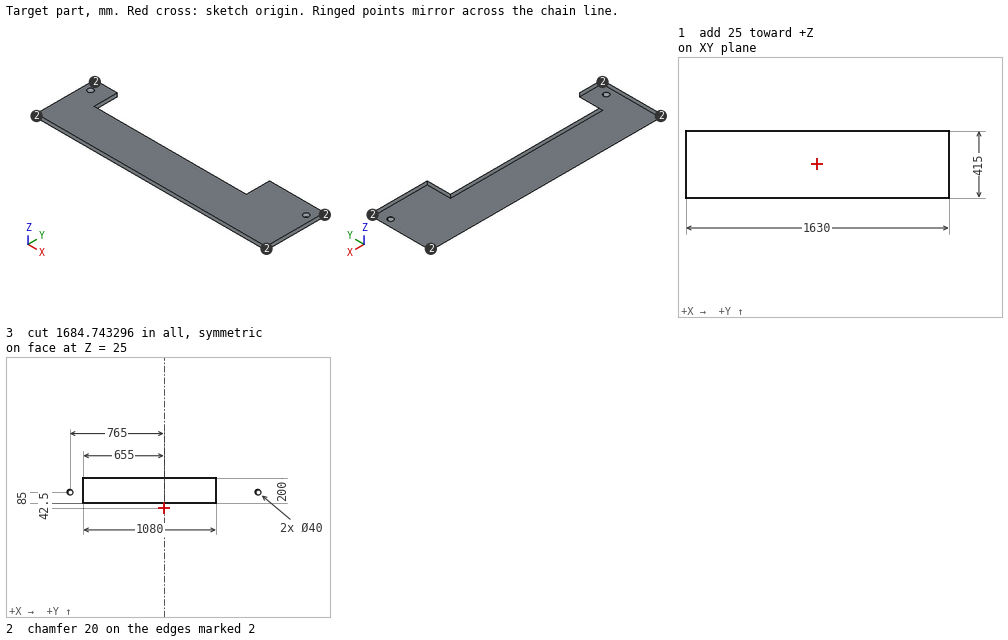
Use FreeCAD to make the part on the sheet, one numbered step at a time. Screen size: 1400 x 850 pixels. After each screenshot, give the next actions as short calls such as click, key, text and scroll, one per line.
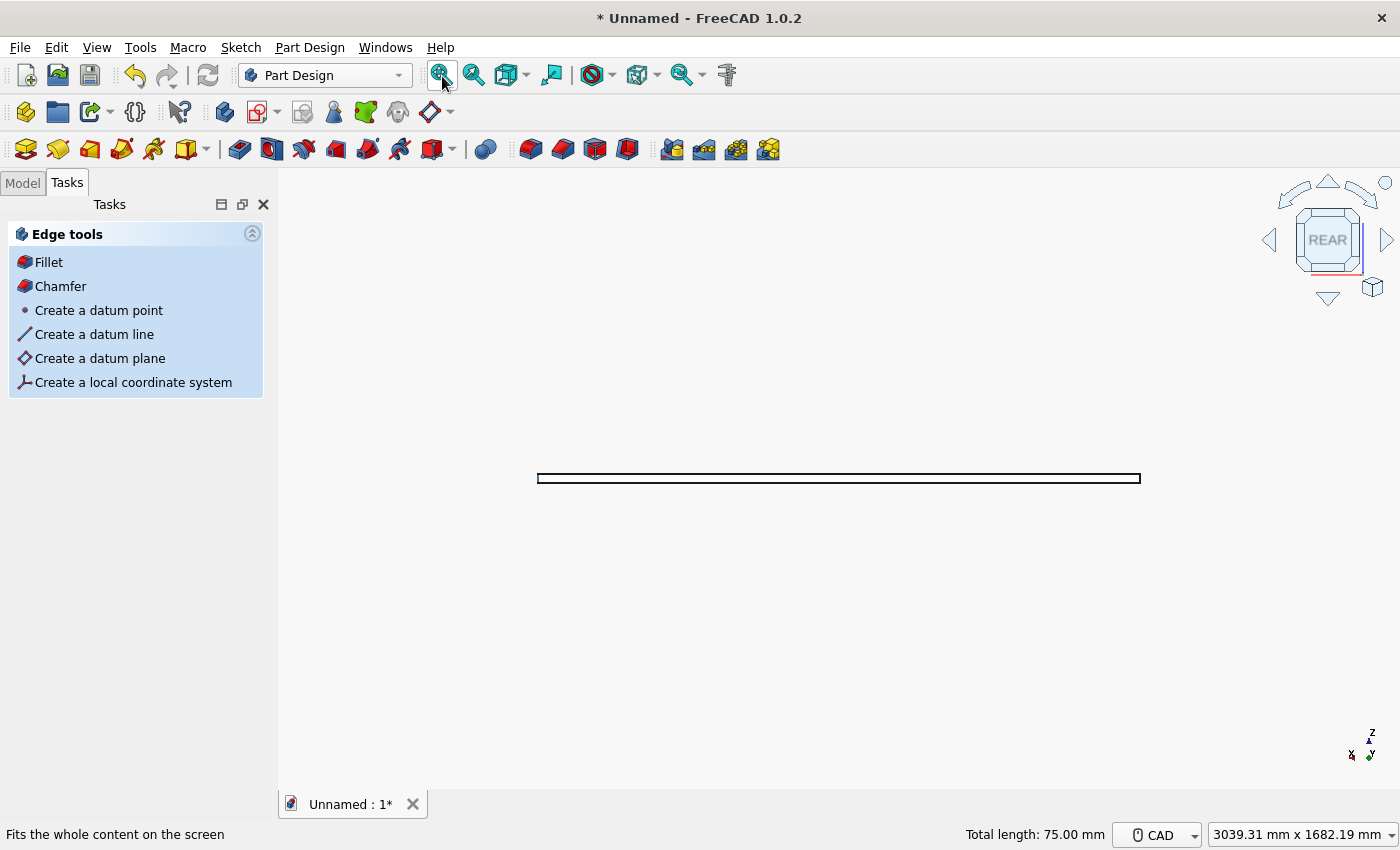
scroll(1140, 478, up, 8)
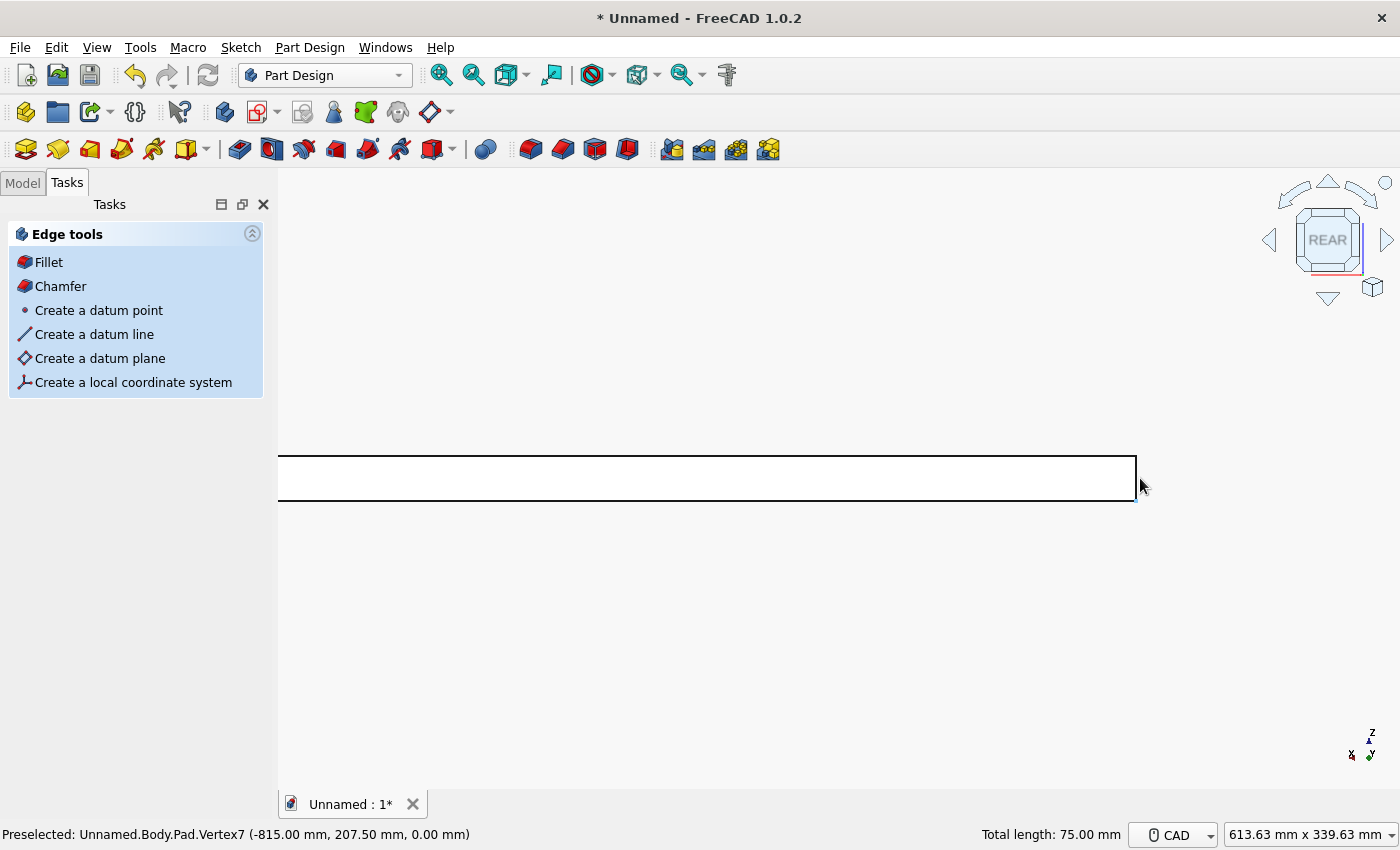
click(1136, 478, ctrl)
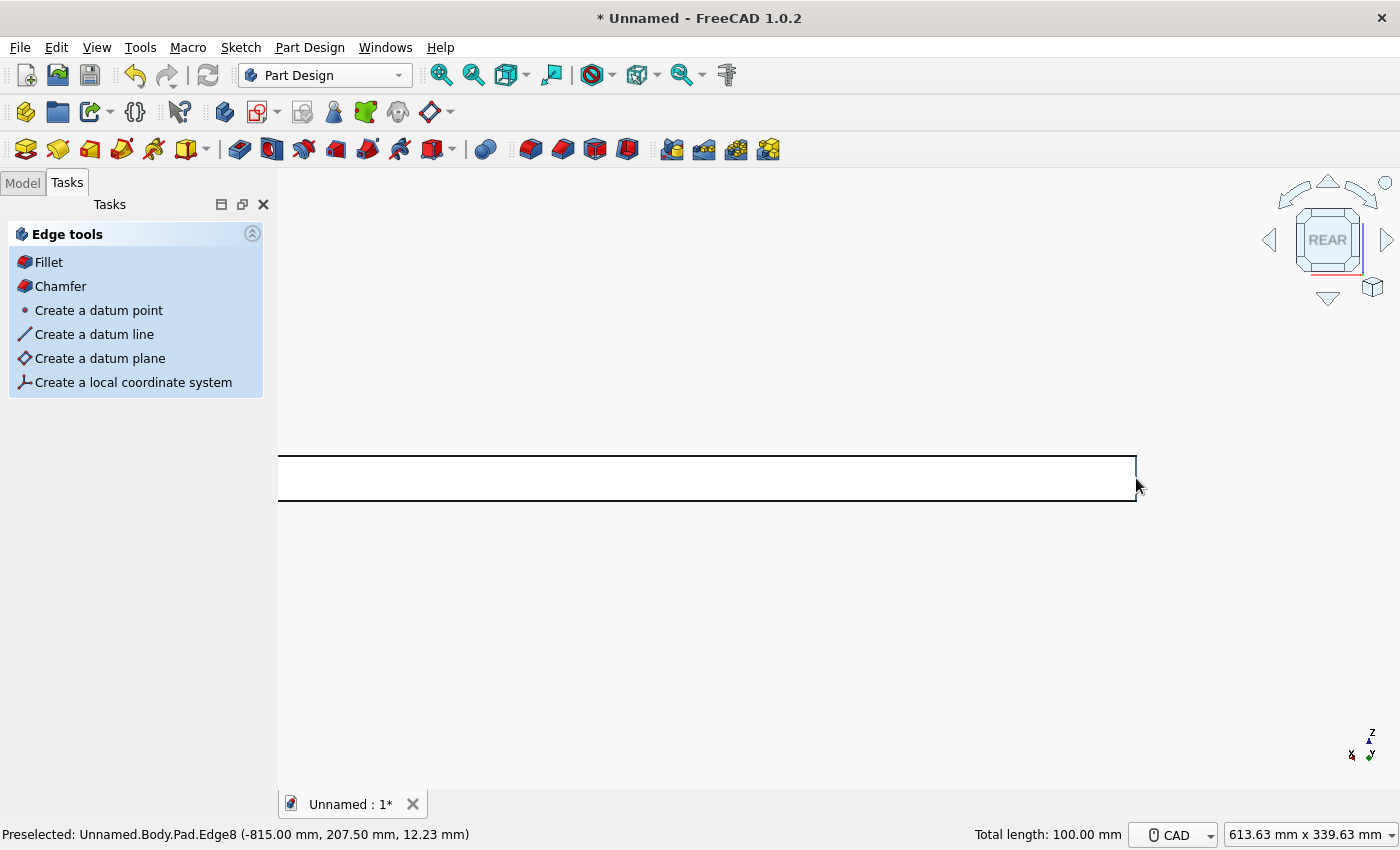
click(564, 150)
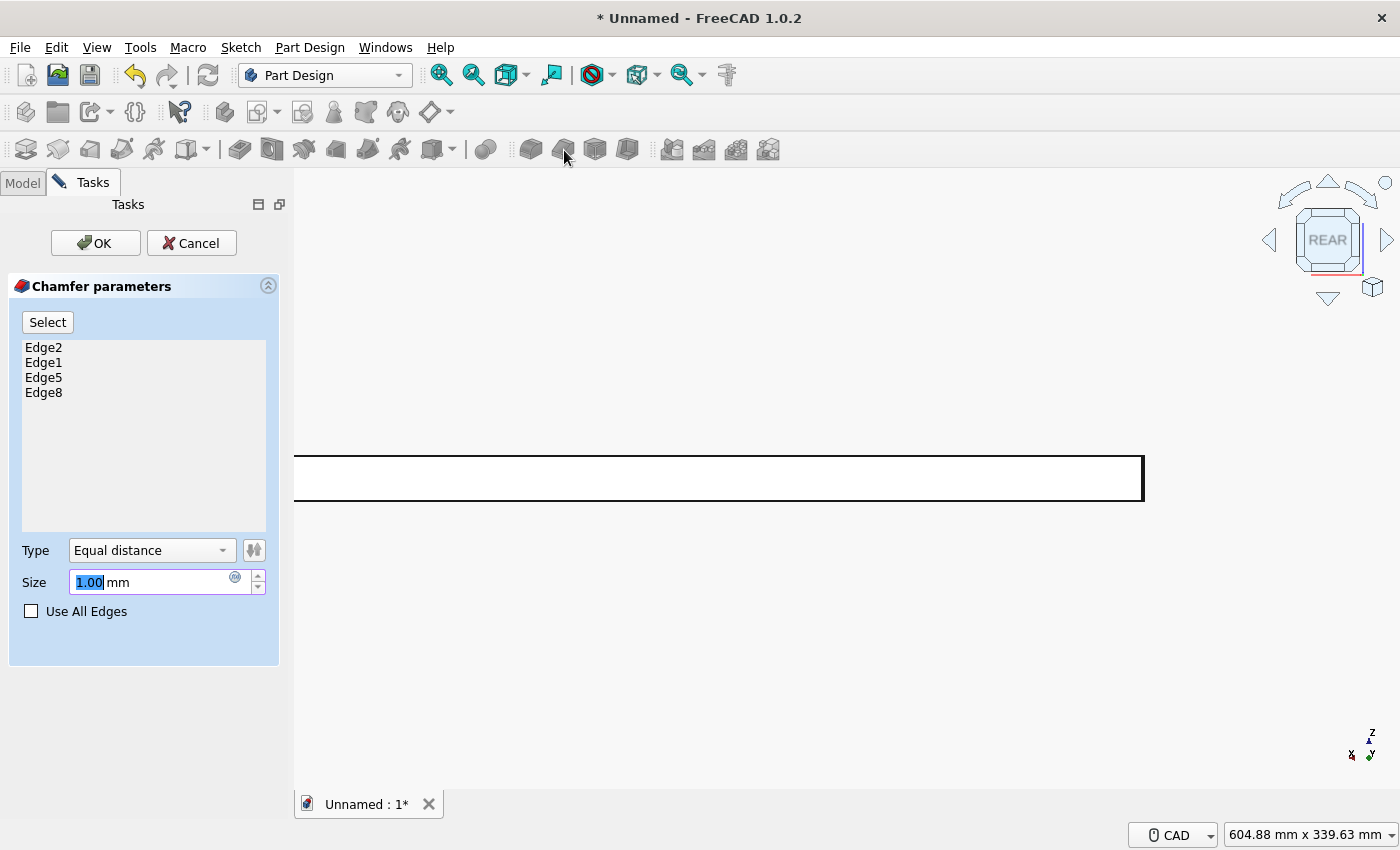
text(20)
key(Tab)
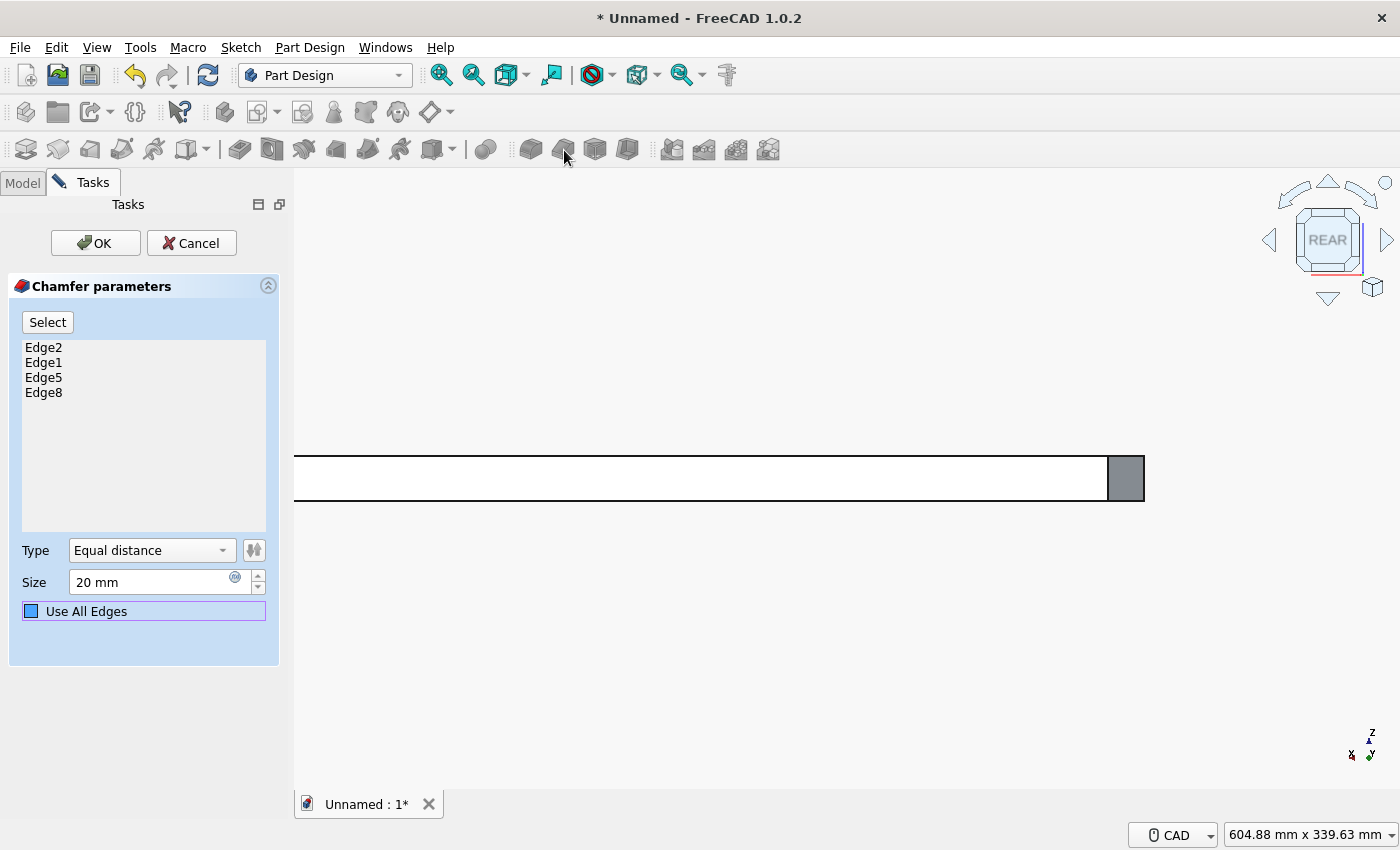
click(96, 243)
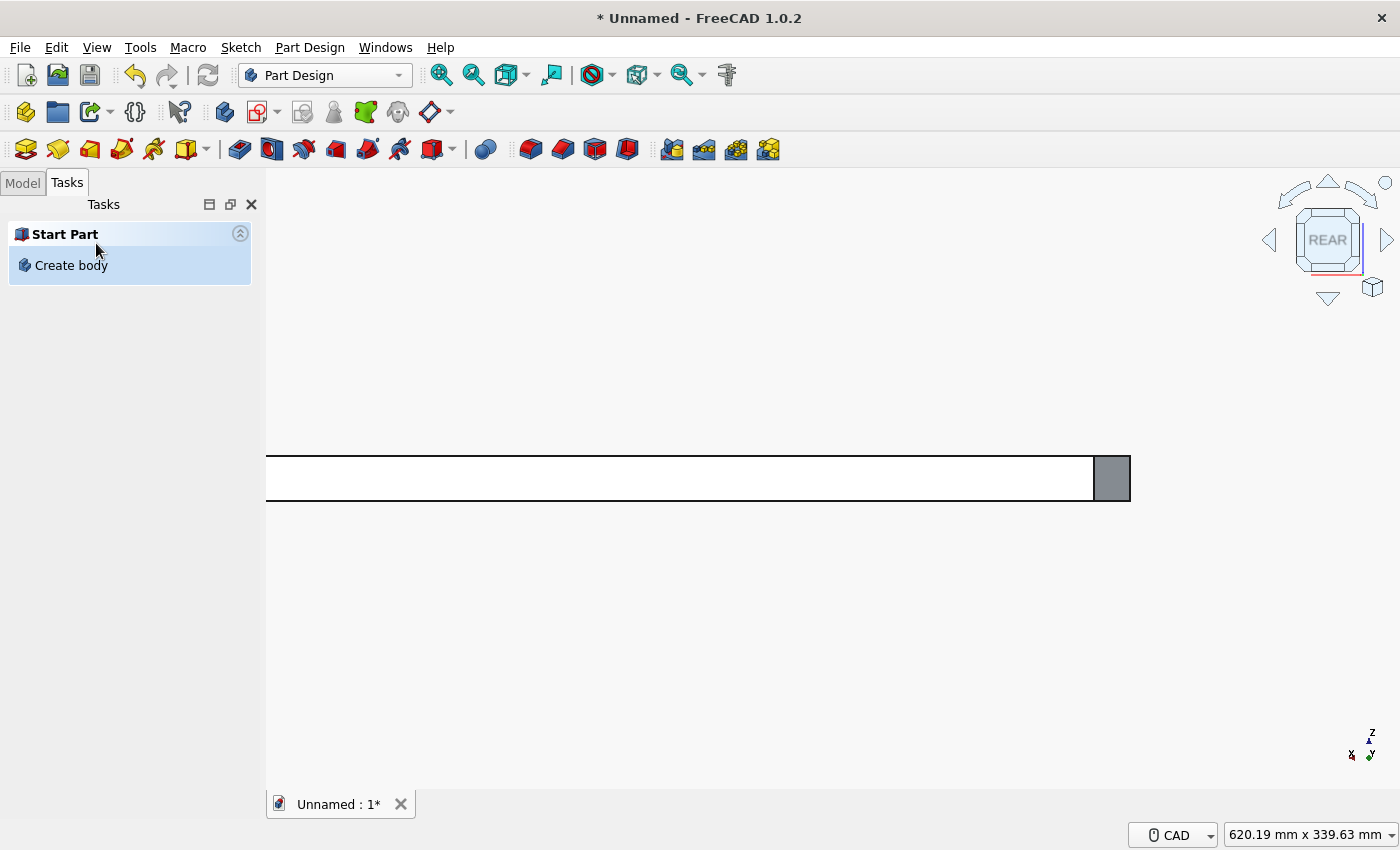
click(442, 76)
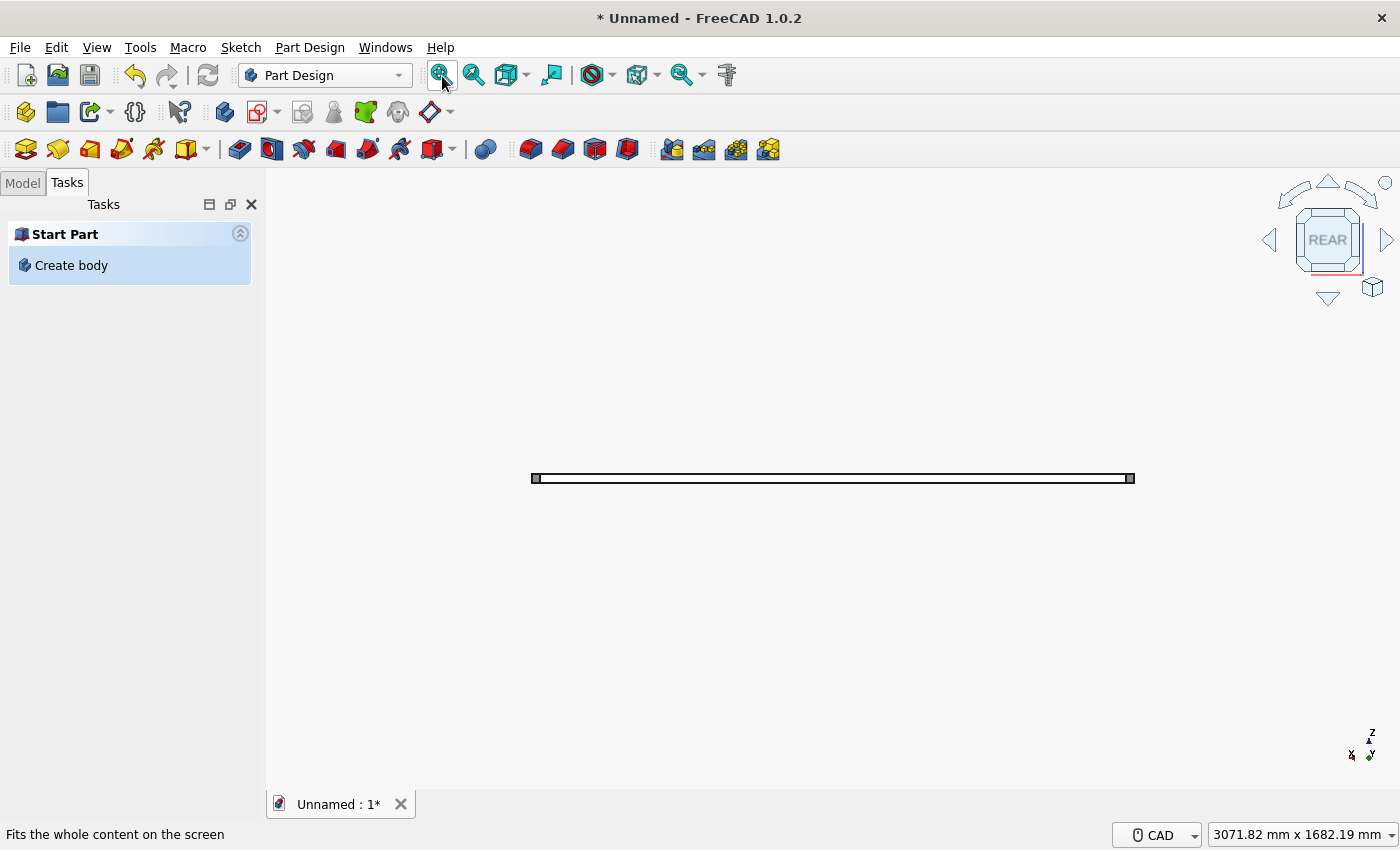
key(0)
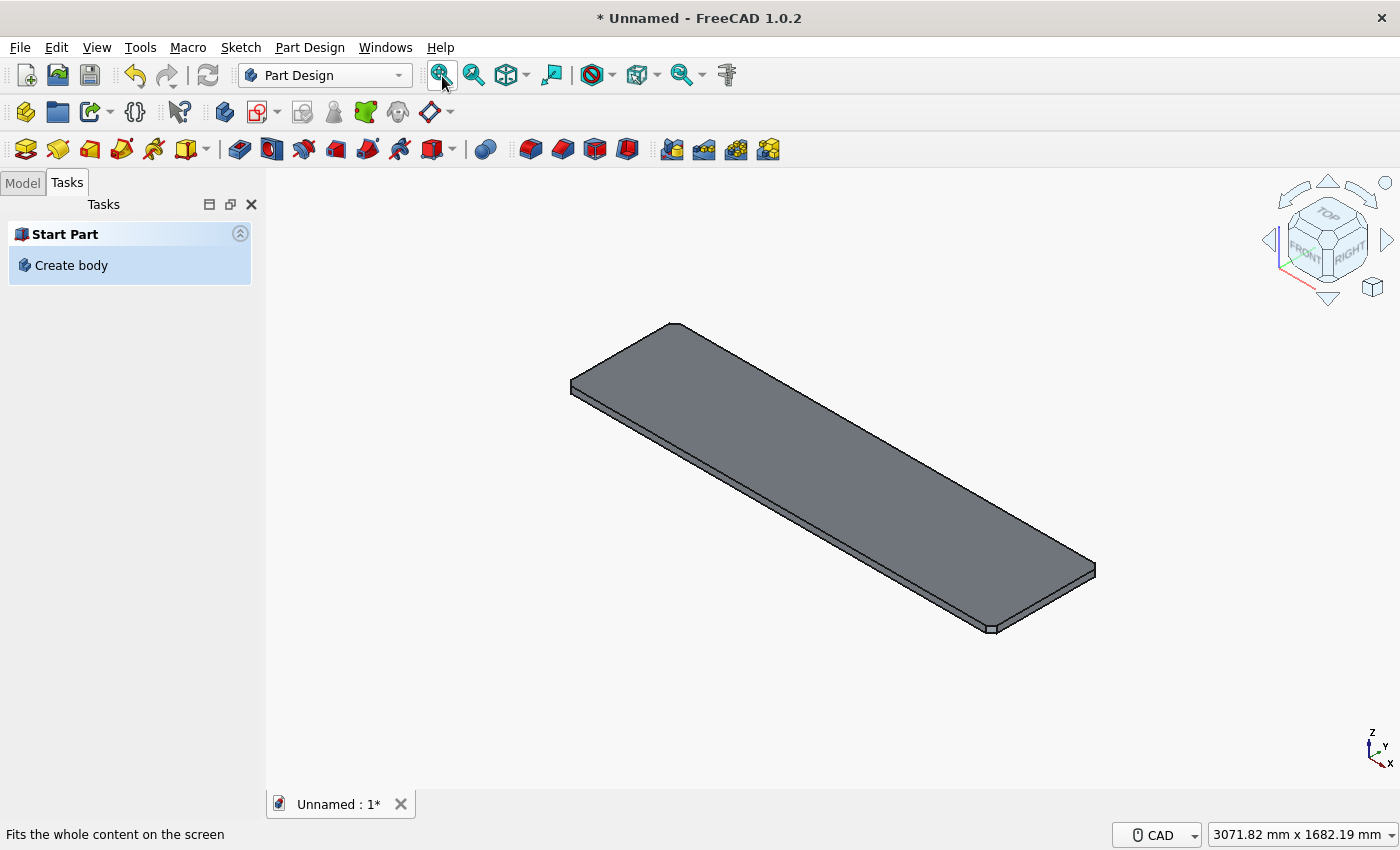
click(955, 544)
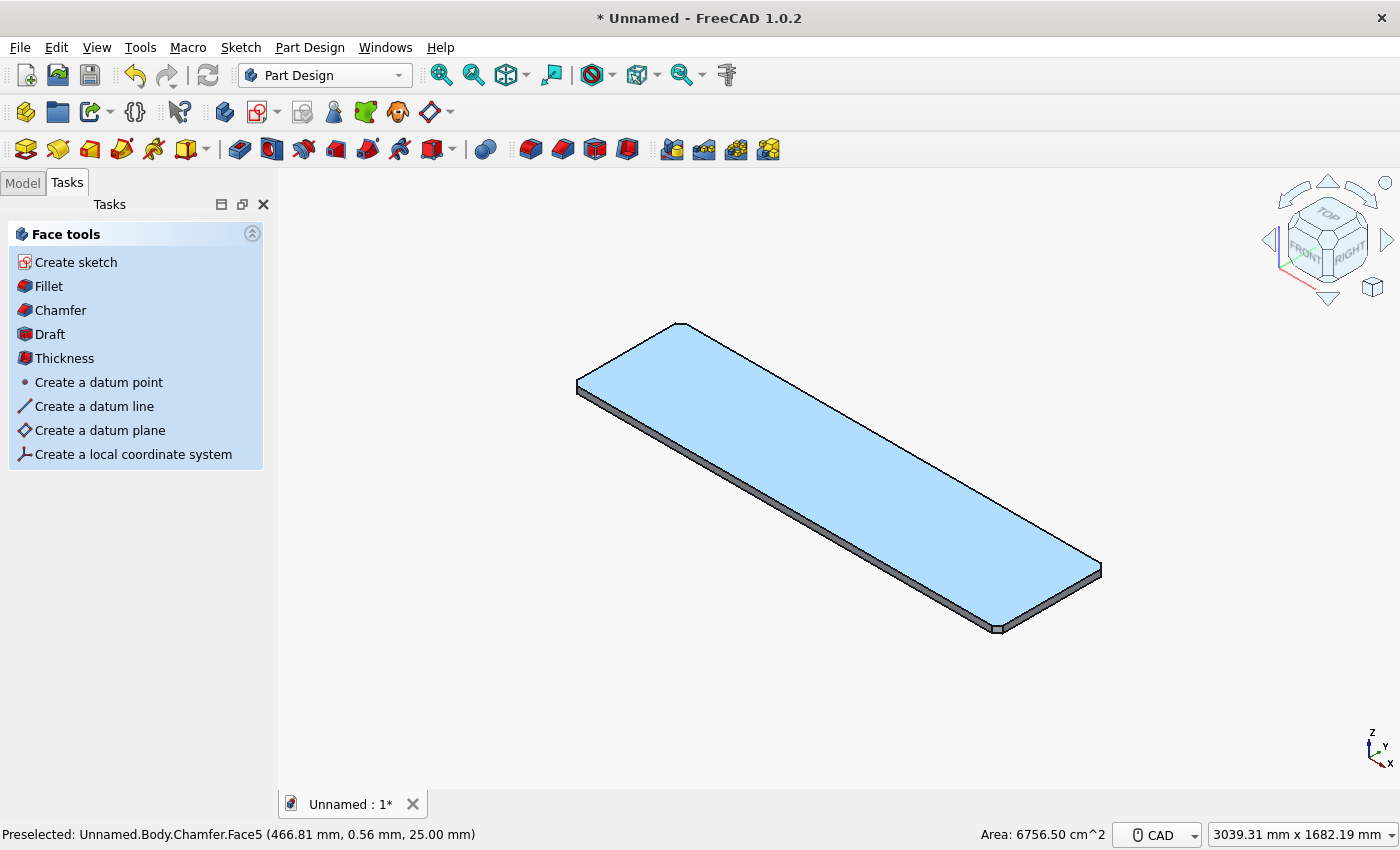
click(258, 112)